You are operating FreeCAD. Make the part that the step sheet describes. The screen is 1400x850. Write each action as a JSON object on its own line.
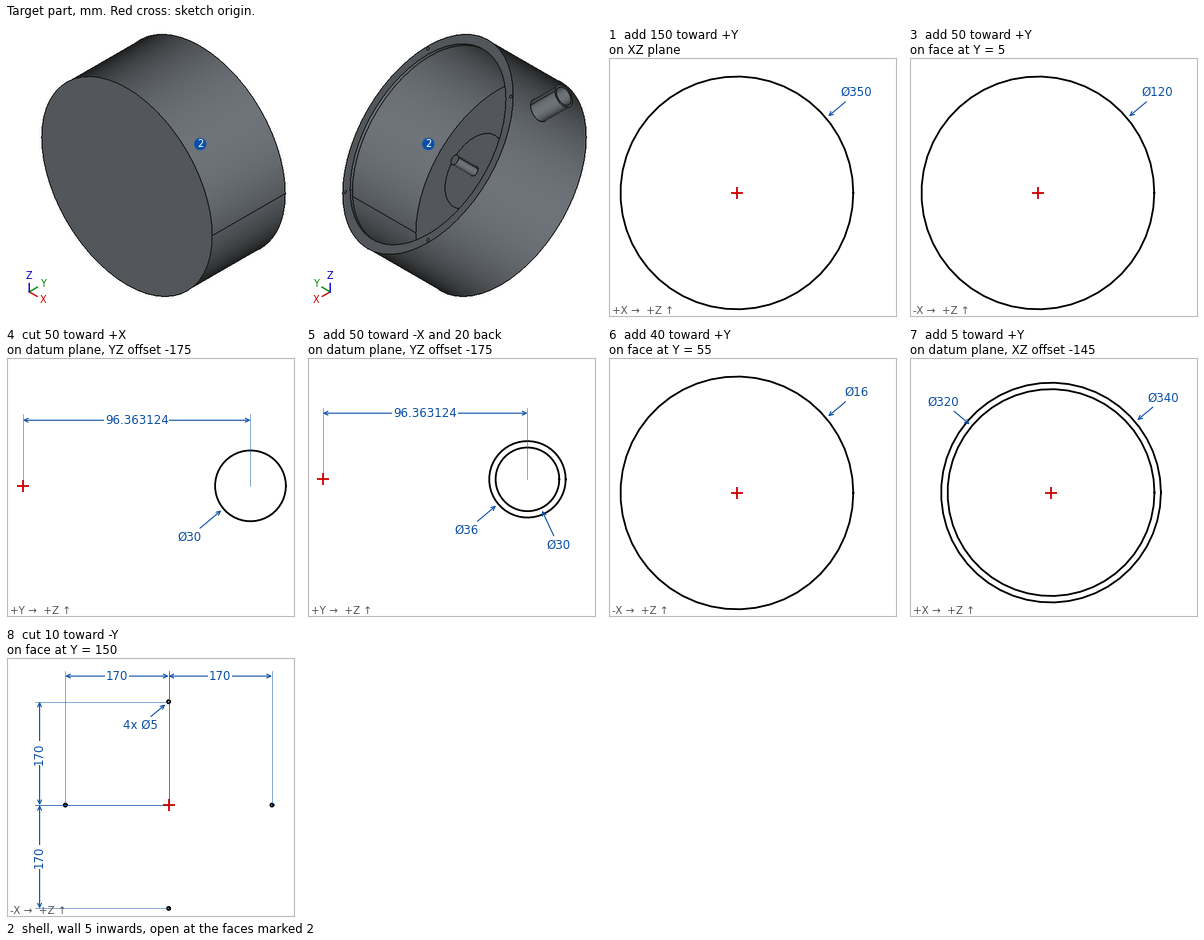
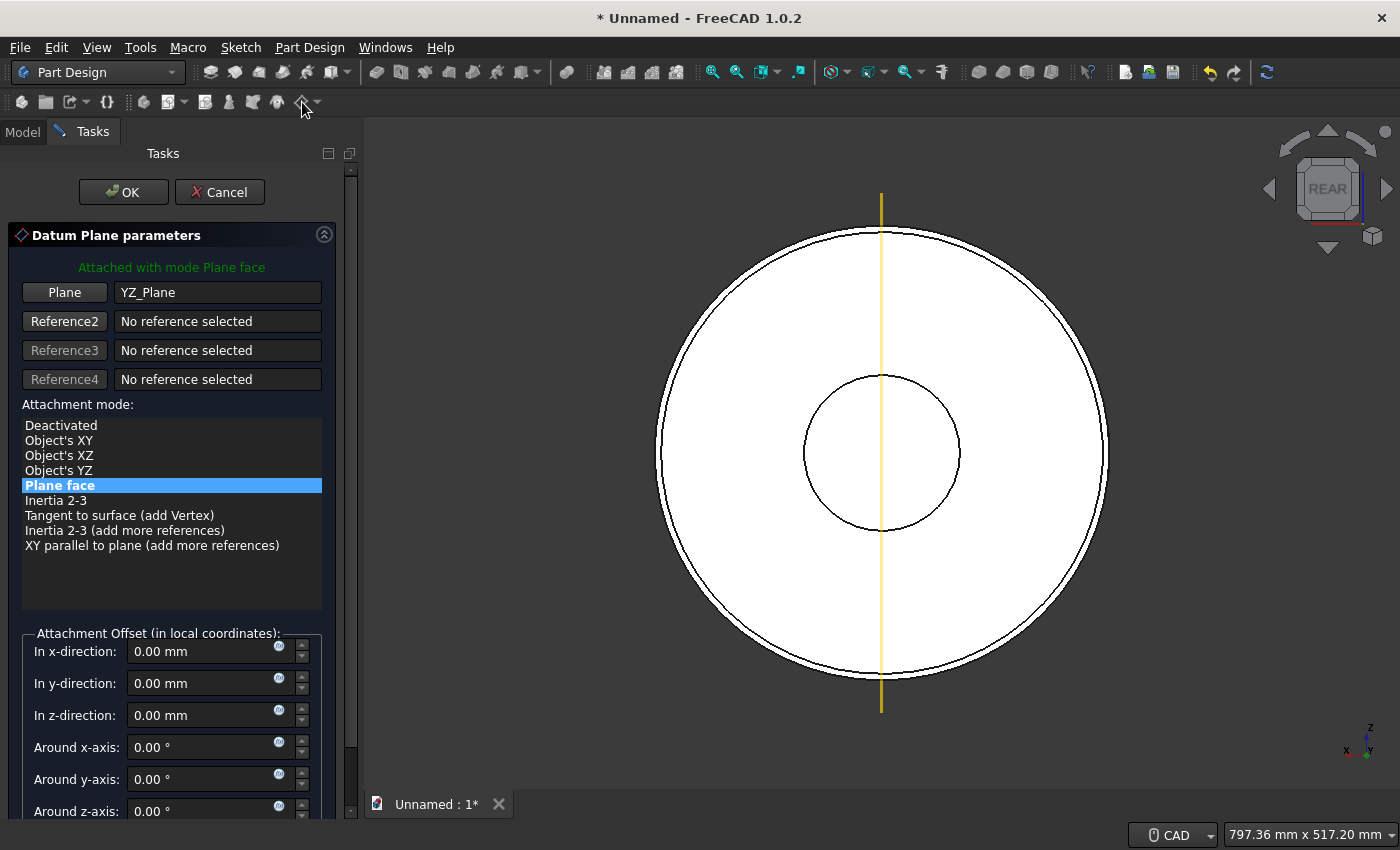
{"action": "triple_click", "coordinate": [210, 715]}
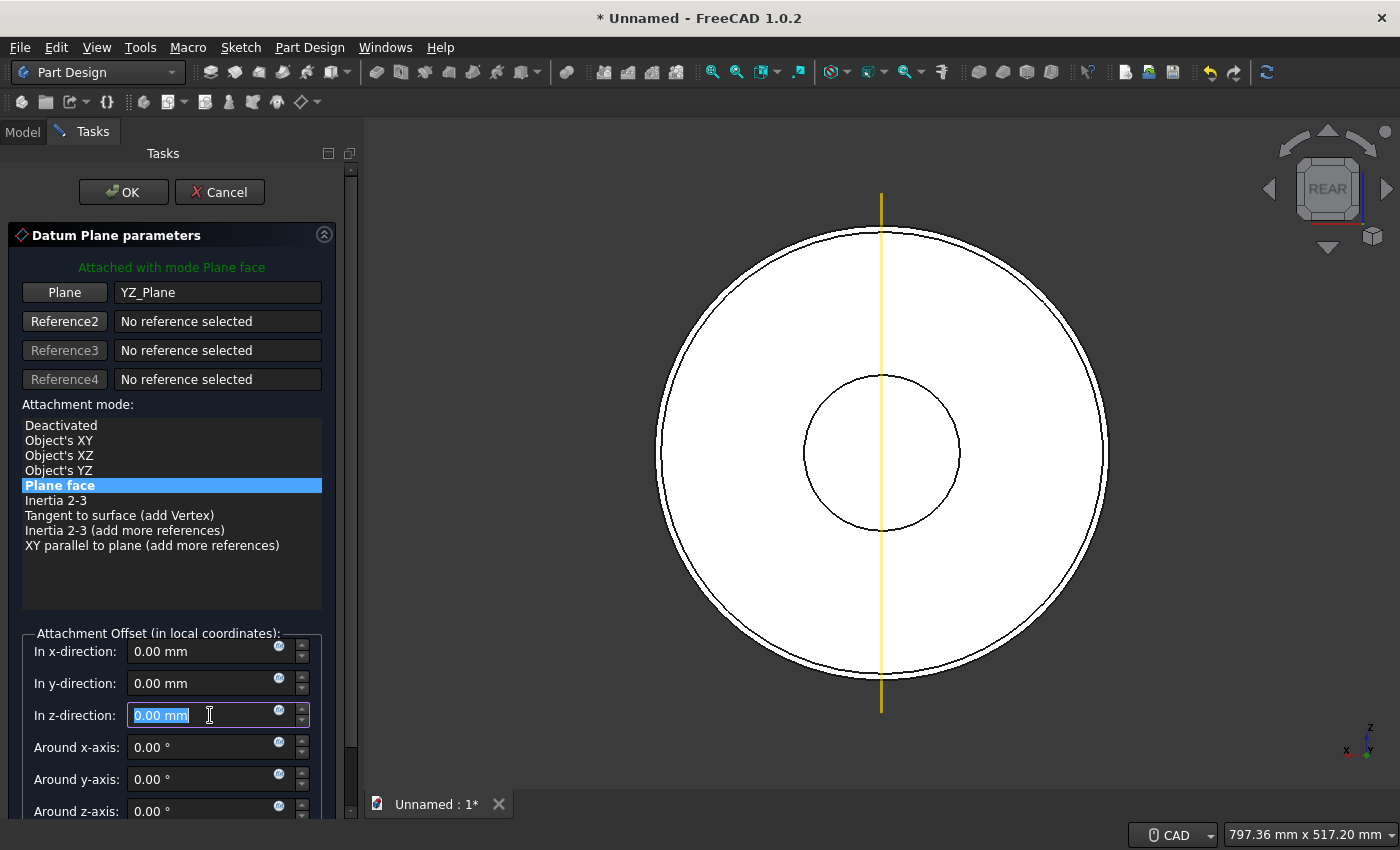
{"action": "type", "text": "-175"}
{"action": "key", "text": "Tab"}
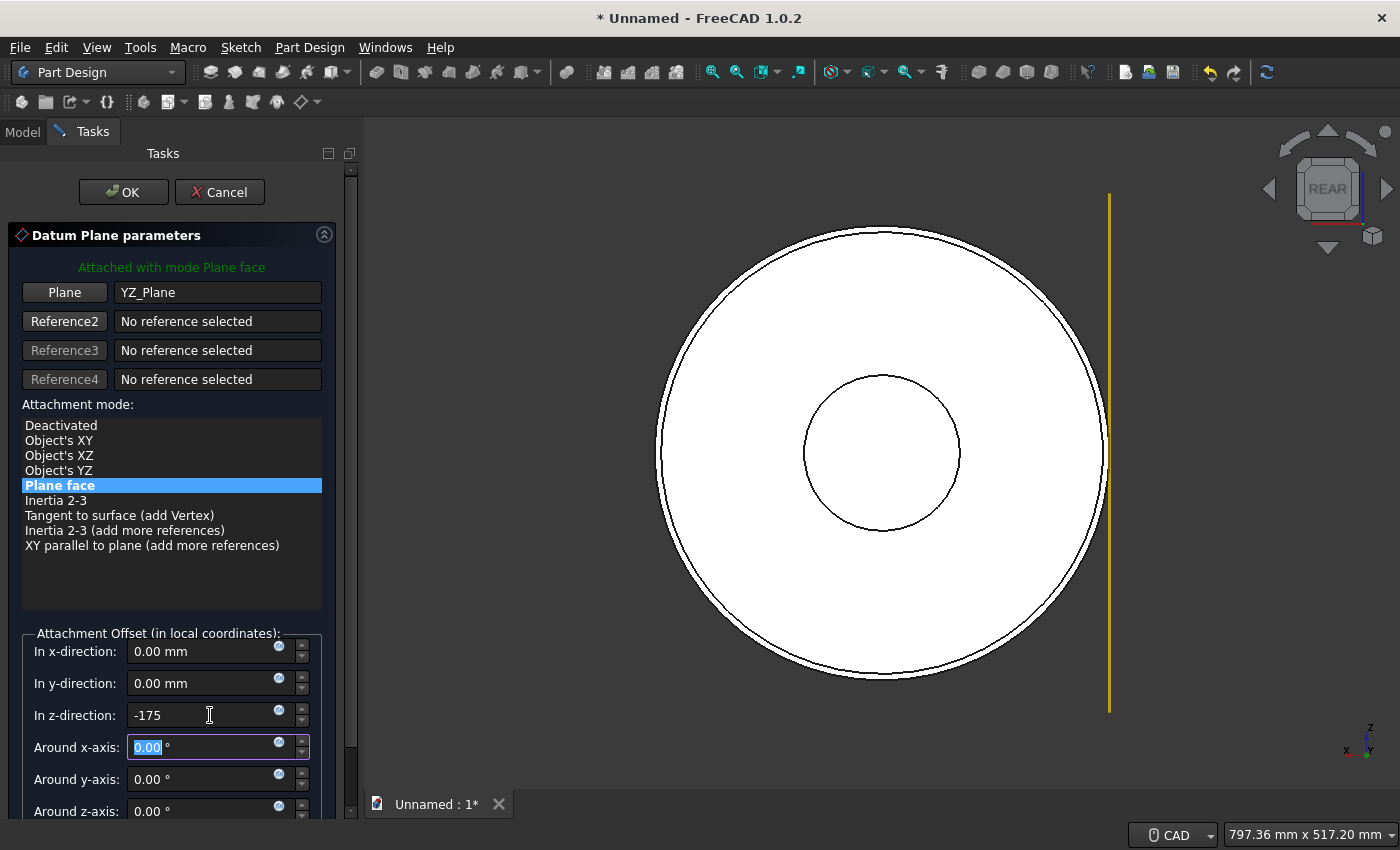
{"action": "left_click", "coordinate": [124, 192]}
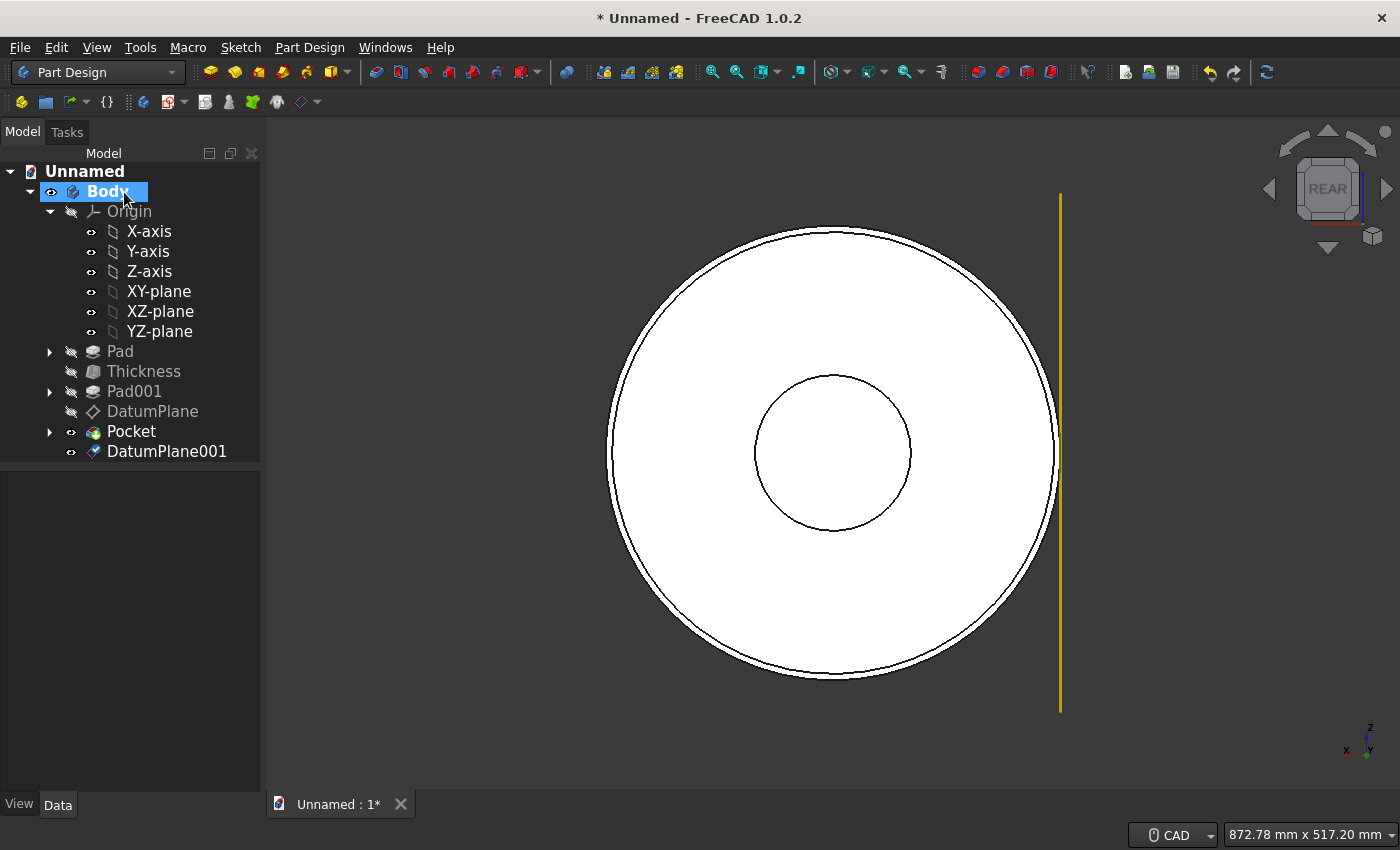
{"action": "left_click", "coordinate": [116, 452]}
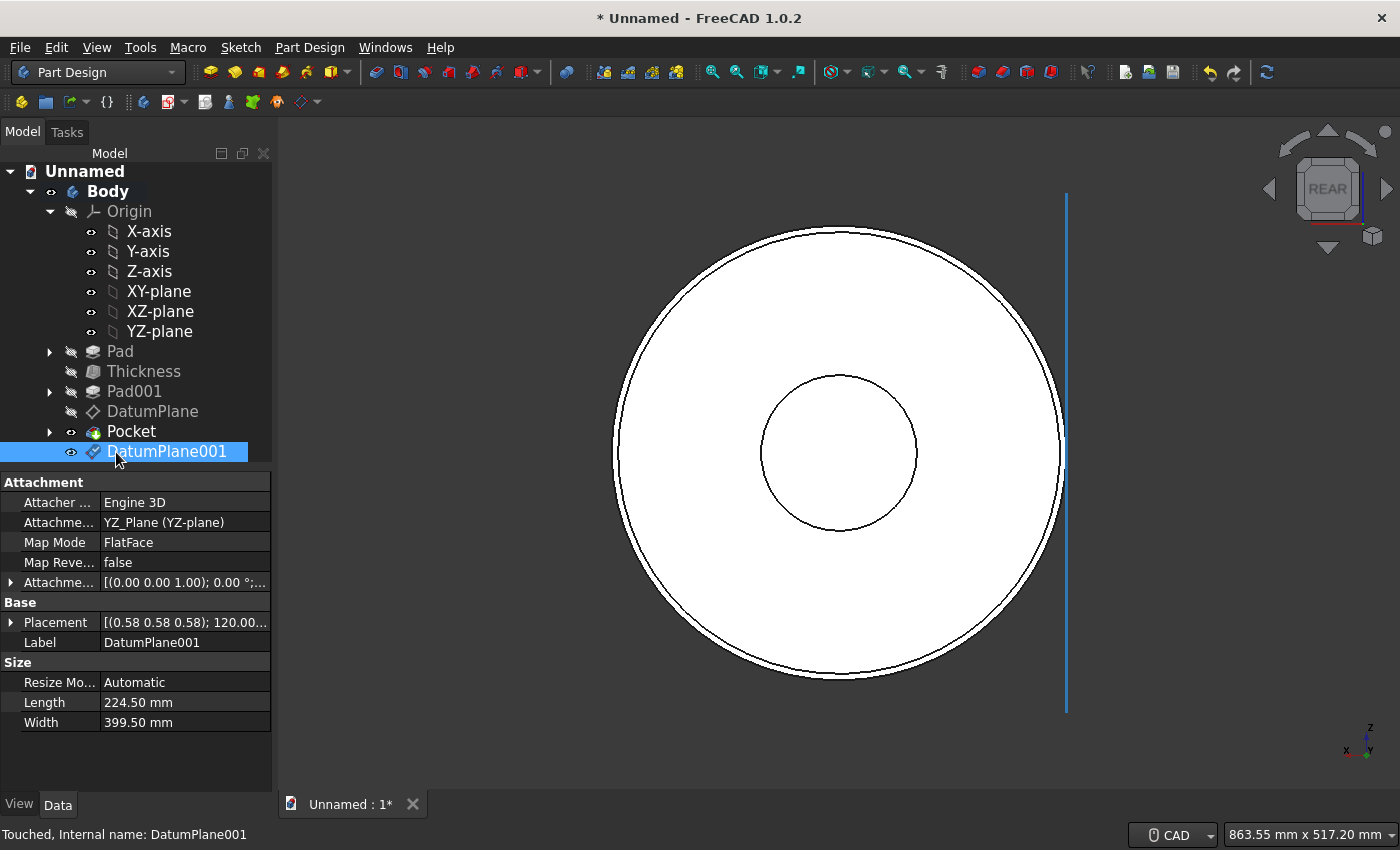
{"action": "left_click", "coordinate": [168, 102]}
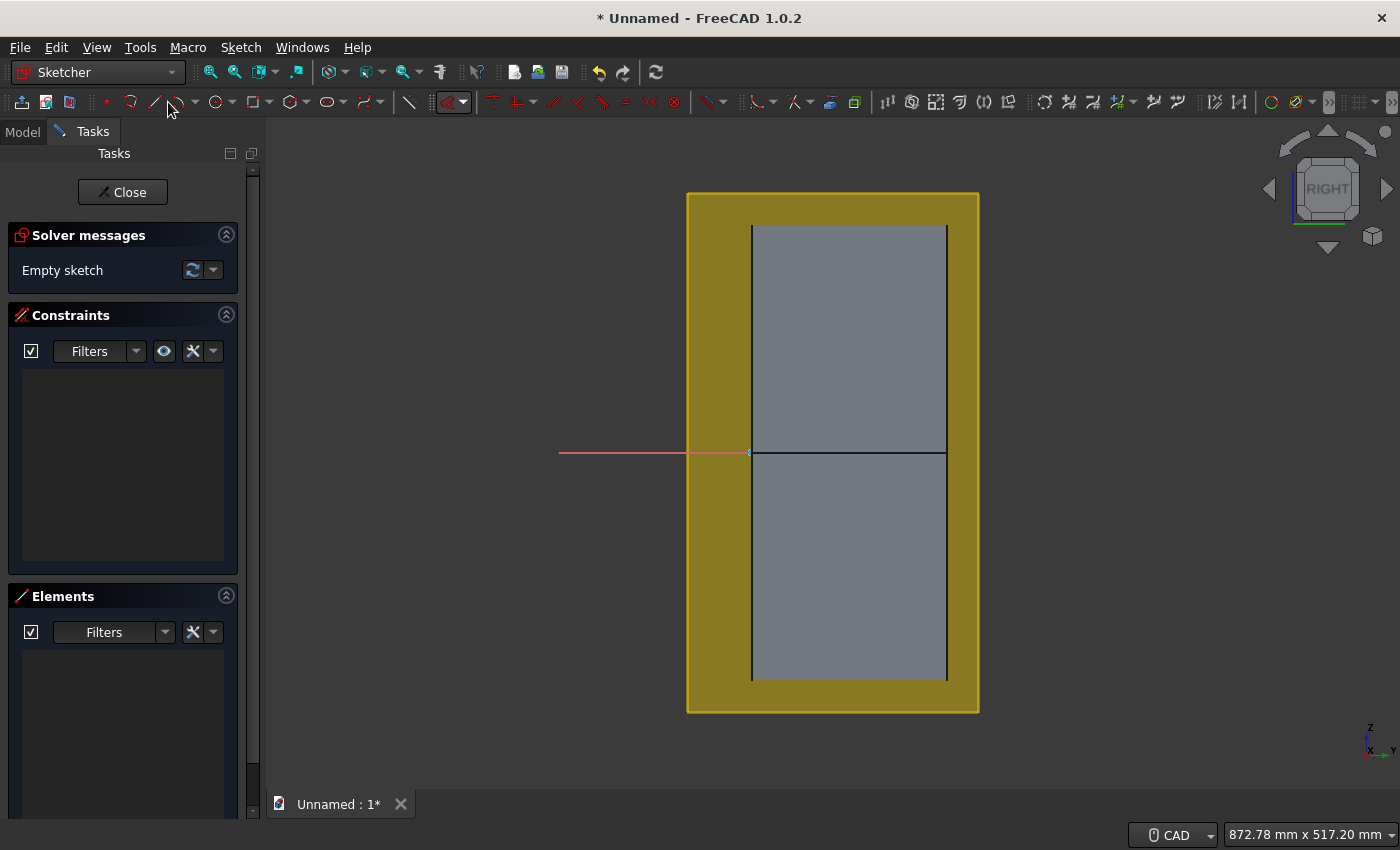
{"action": "left_click", "coordinate": [70, 102]}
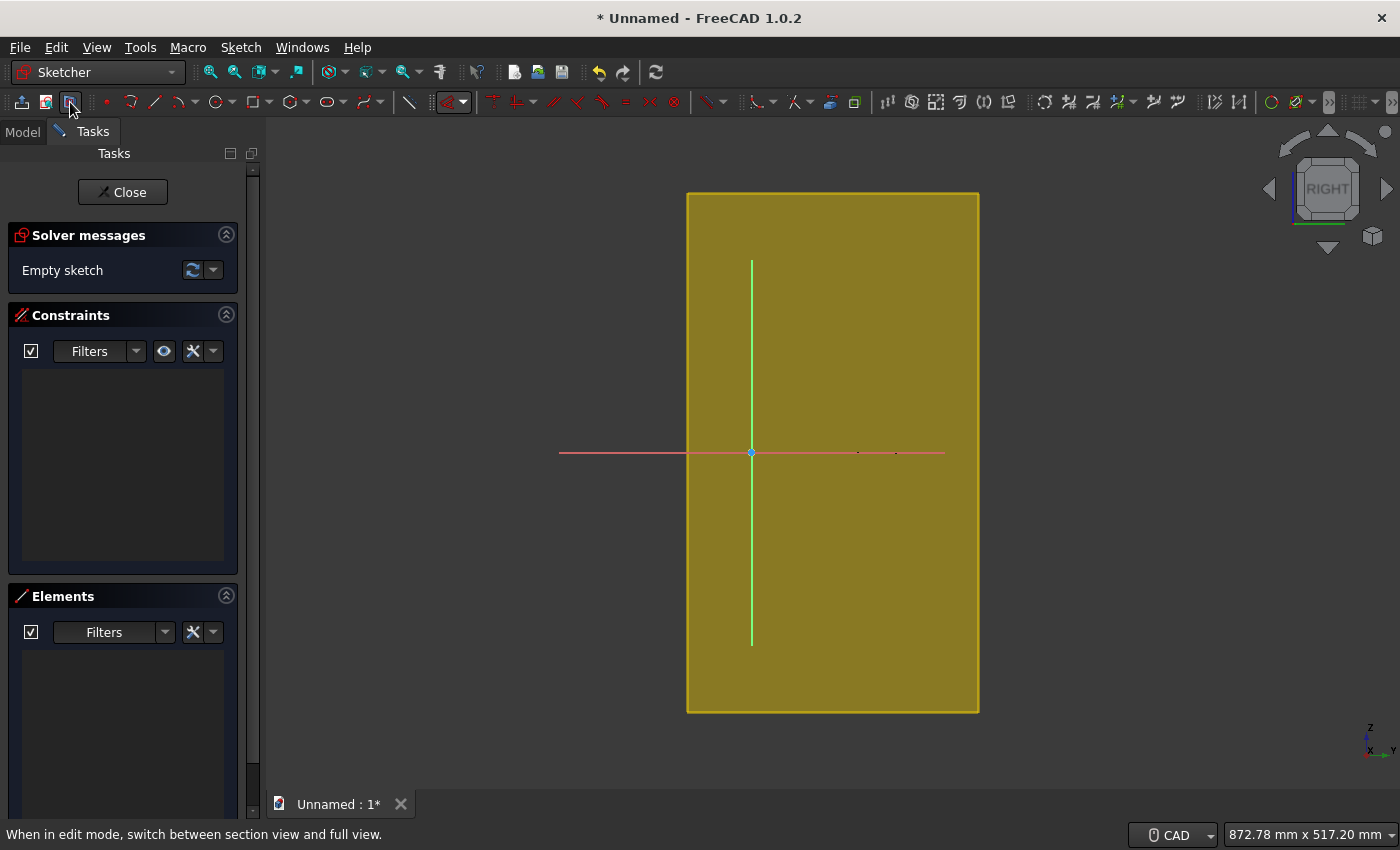
{"action": "scroll", "coordinate": [891, 453], "scroll_direction": "up", "scroll_amount": 11}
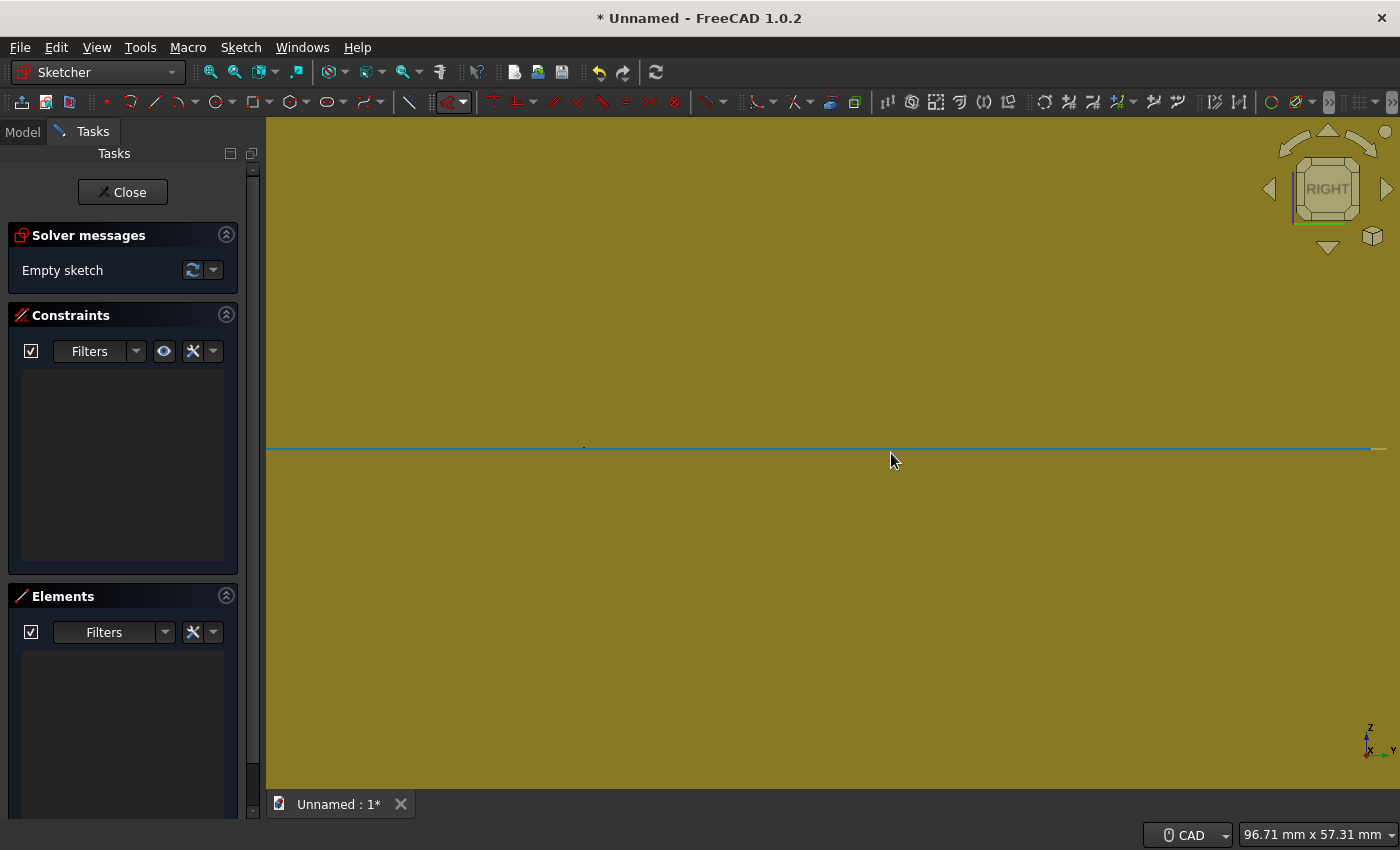
{"action": "left_click", "coordinate": [216, 102]}